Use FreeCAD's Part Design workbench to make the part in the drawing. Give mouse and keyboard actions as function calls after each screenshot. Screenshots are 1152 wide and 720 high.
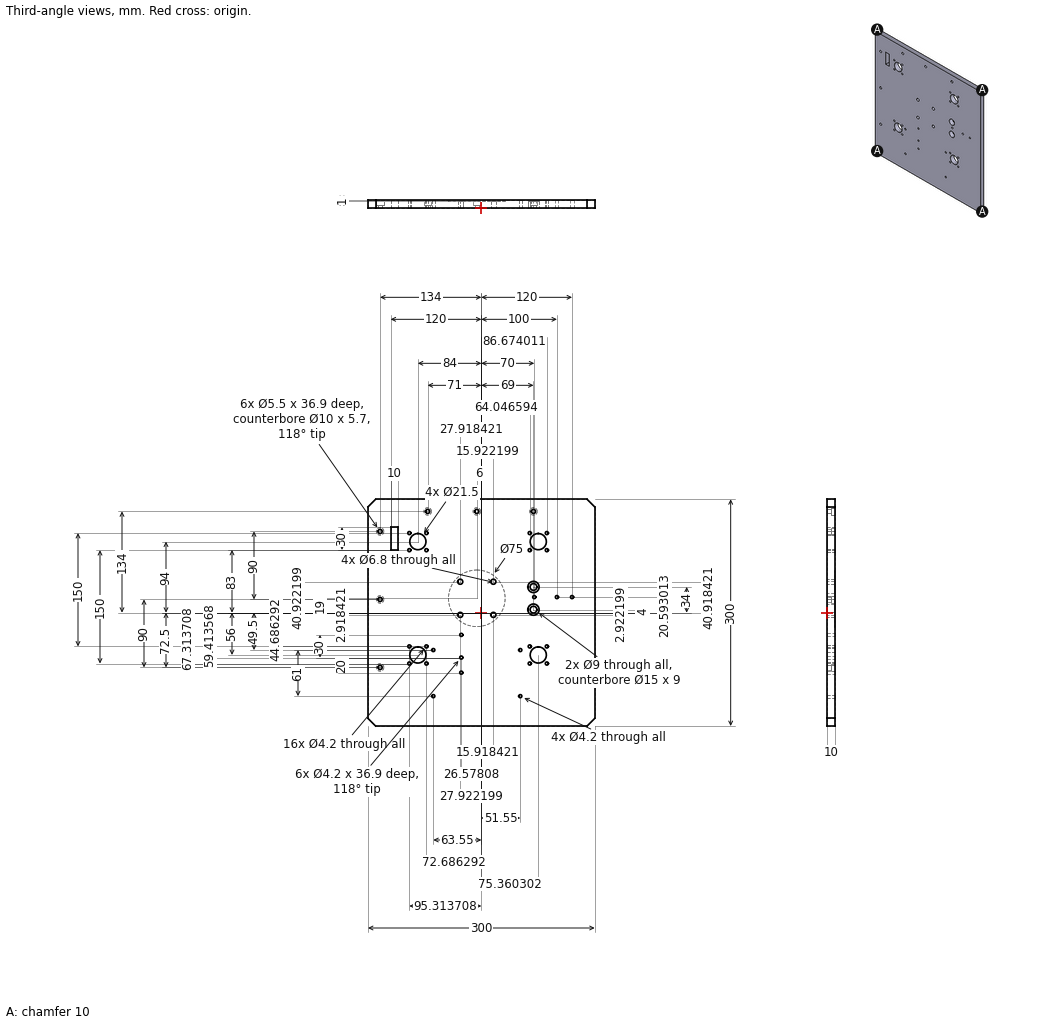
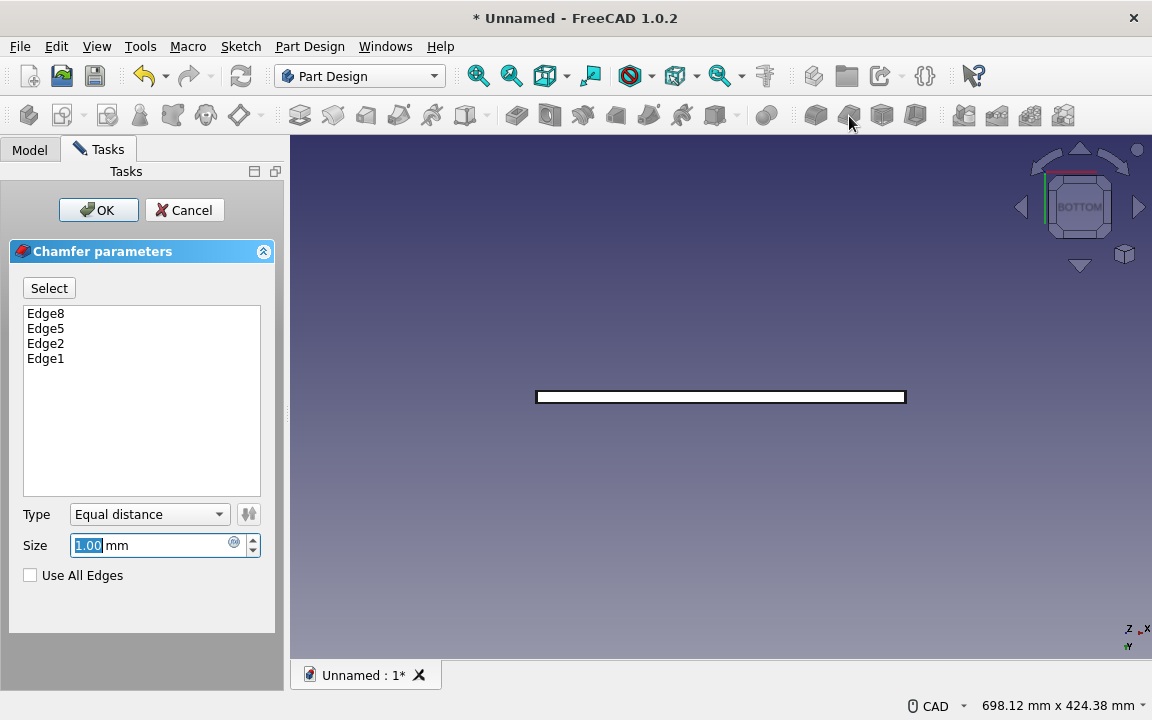
text(10)
key(Tab)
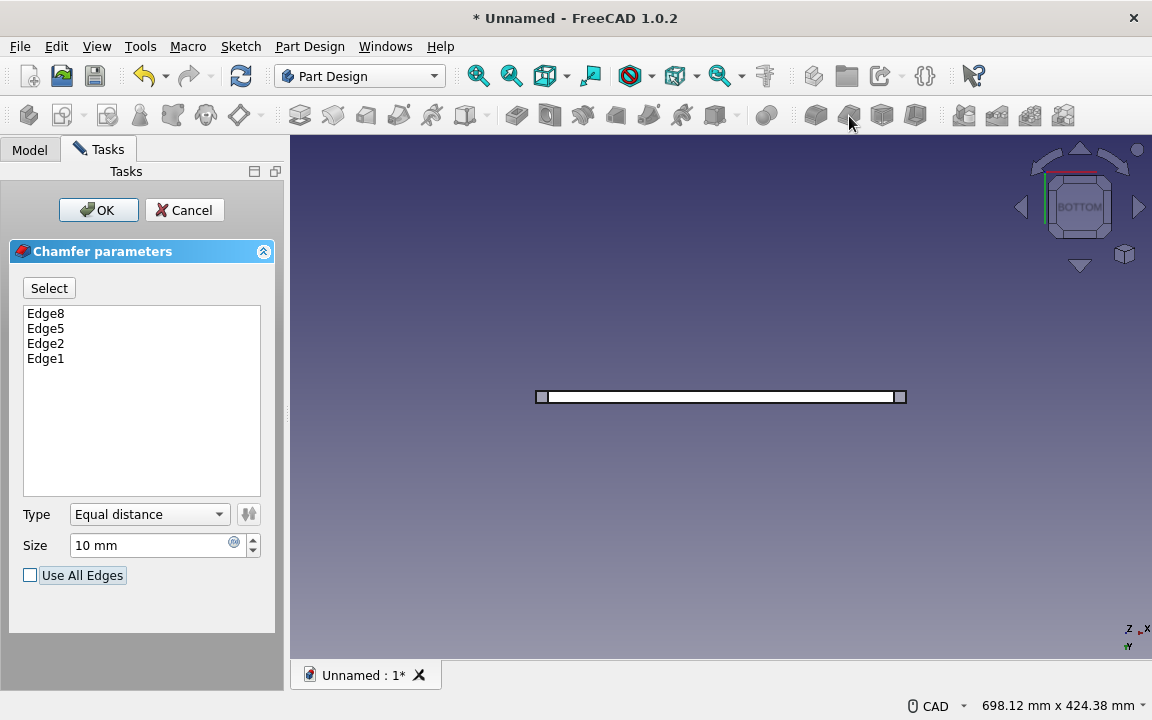
click(99, 210)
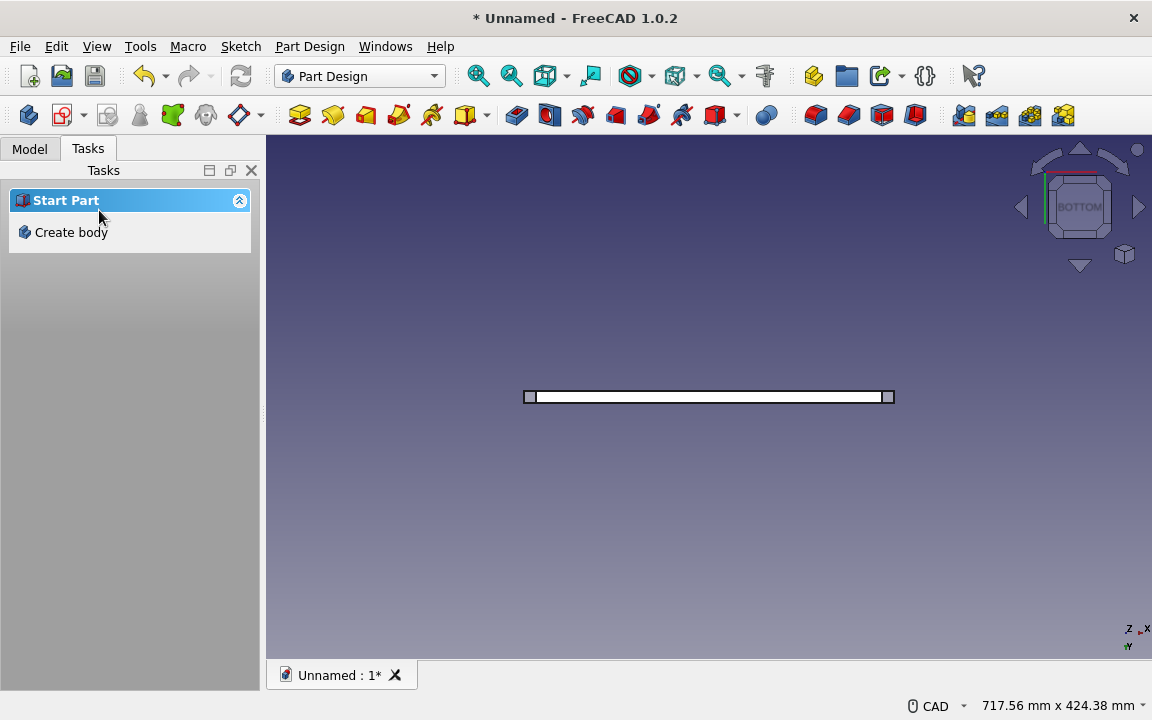
click(479, 76)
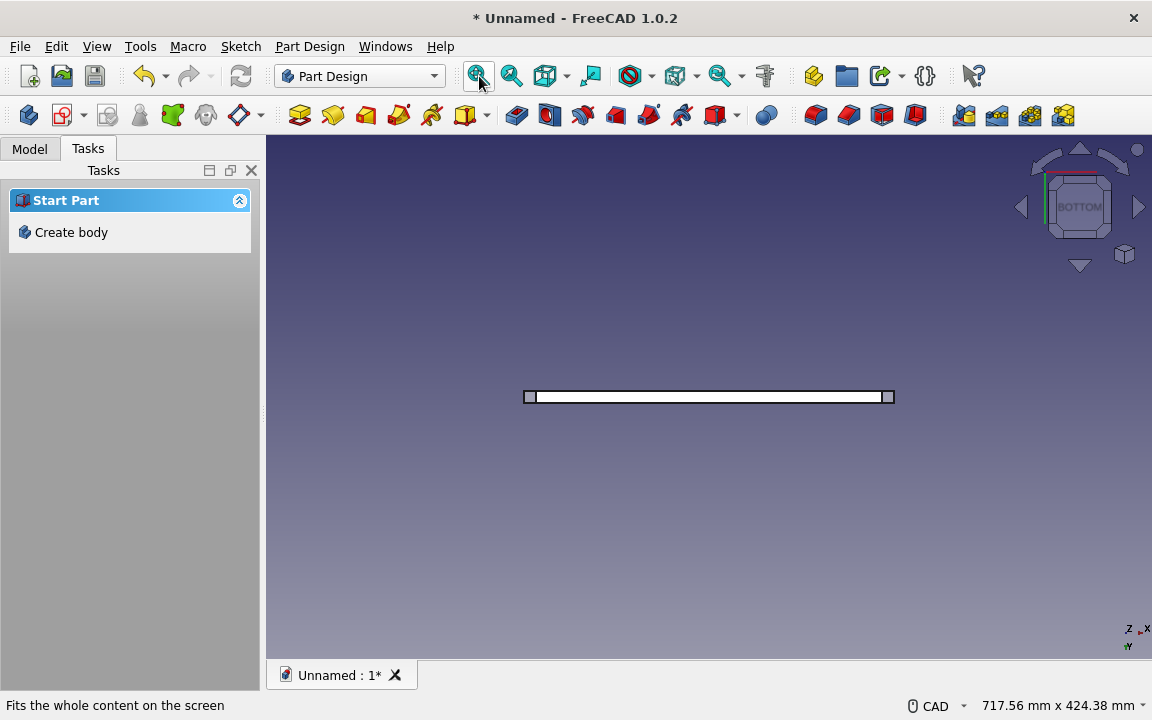
key(0)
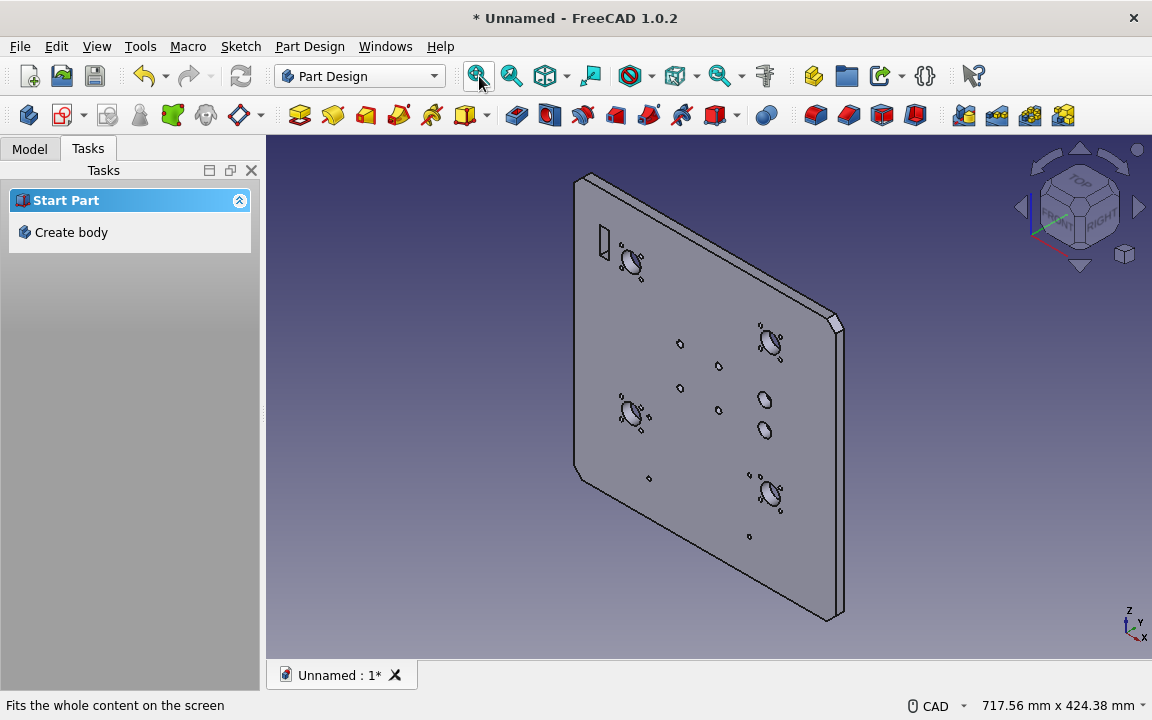
click(705, 485)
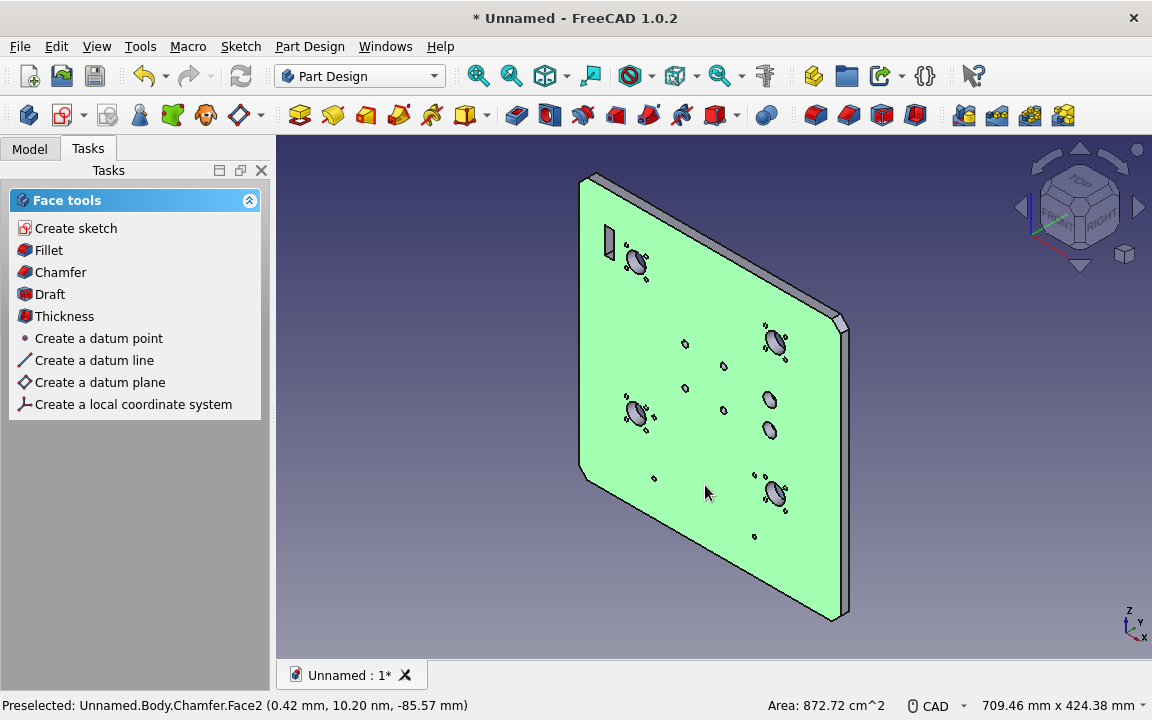
click(62, 116)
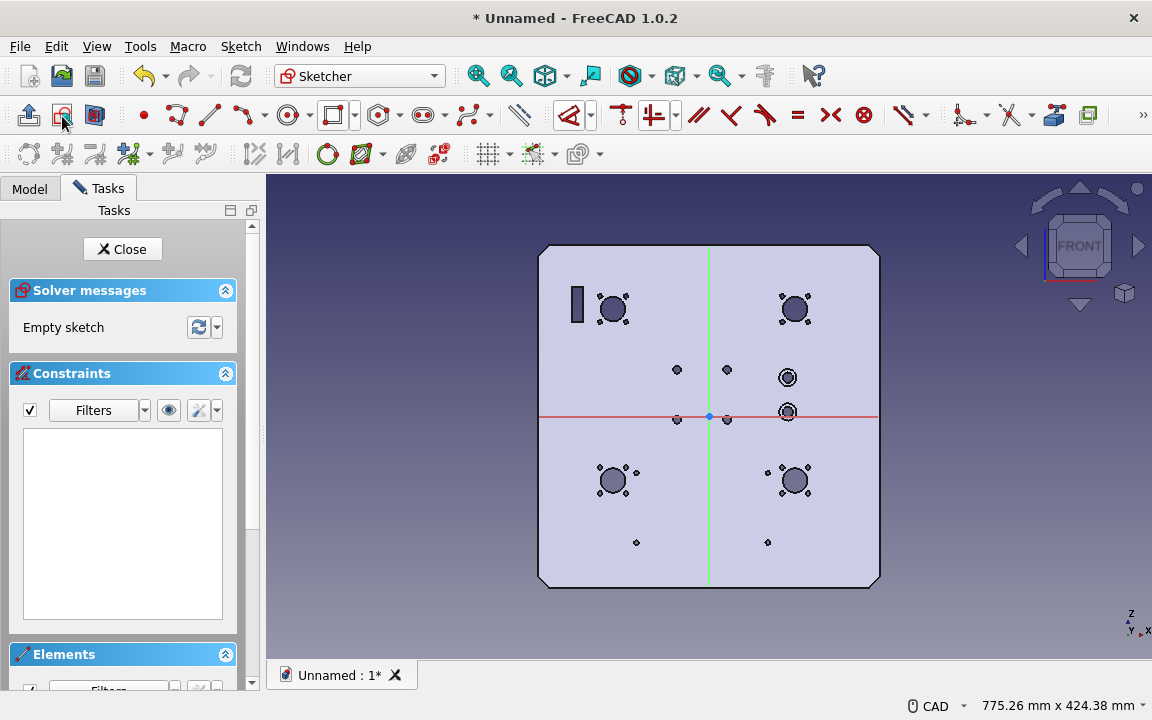
scroll(833, 470, up, 5)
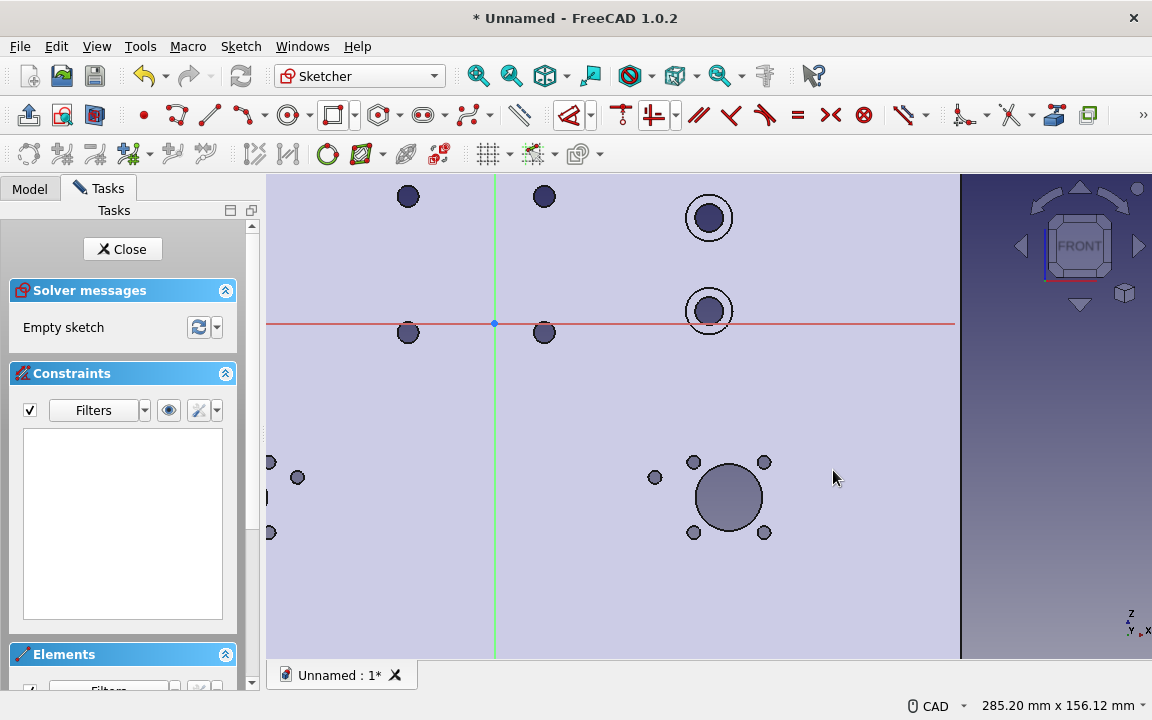
key(g)
key(c)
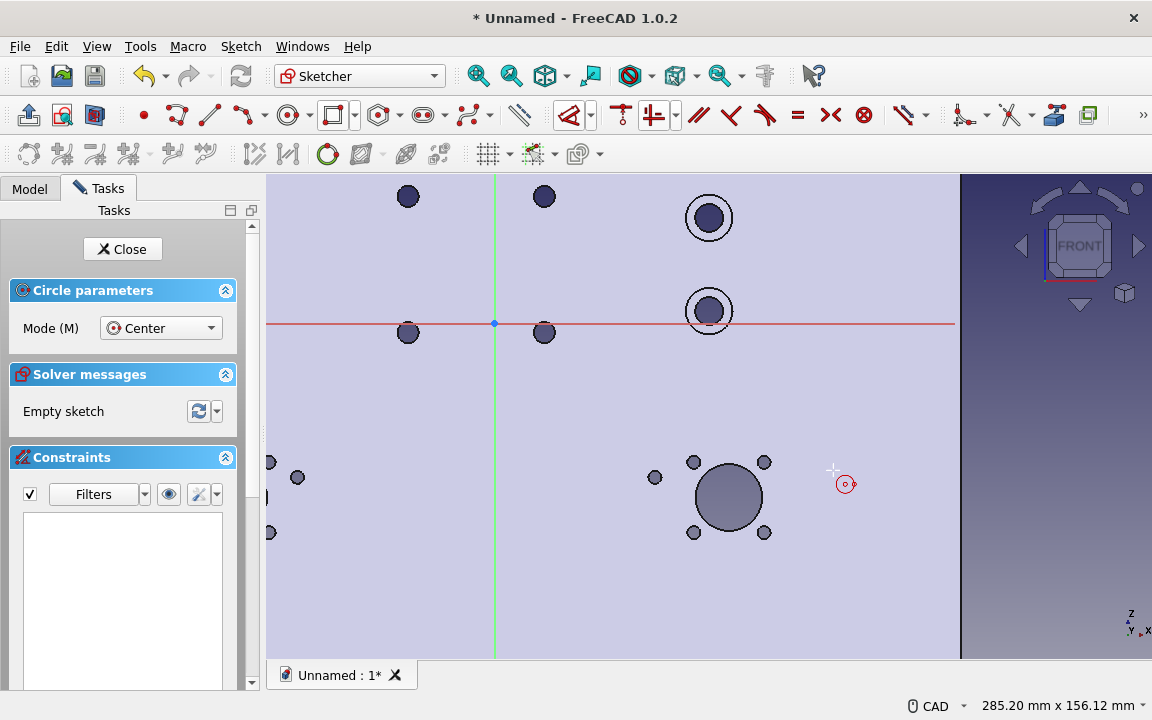
scroll(412, 508, up, 7)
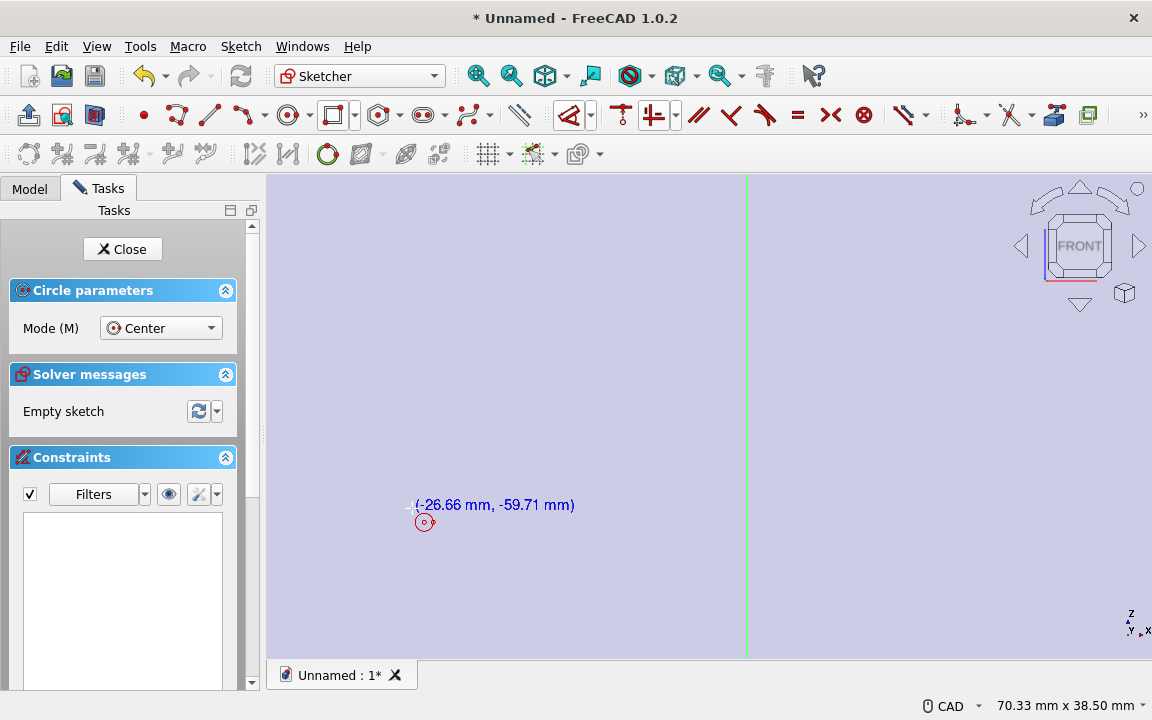
scroll(413, 511, down, 7)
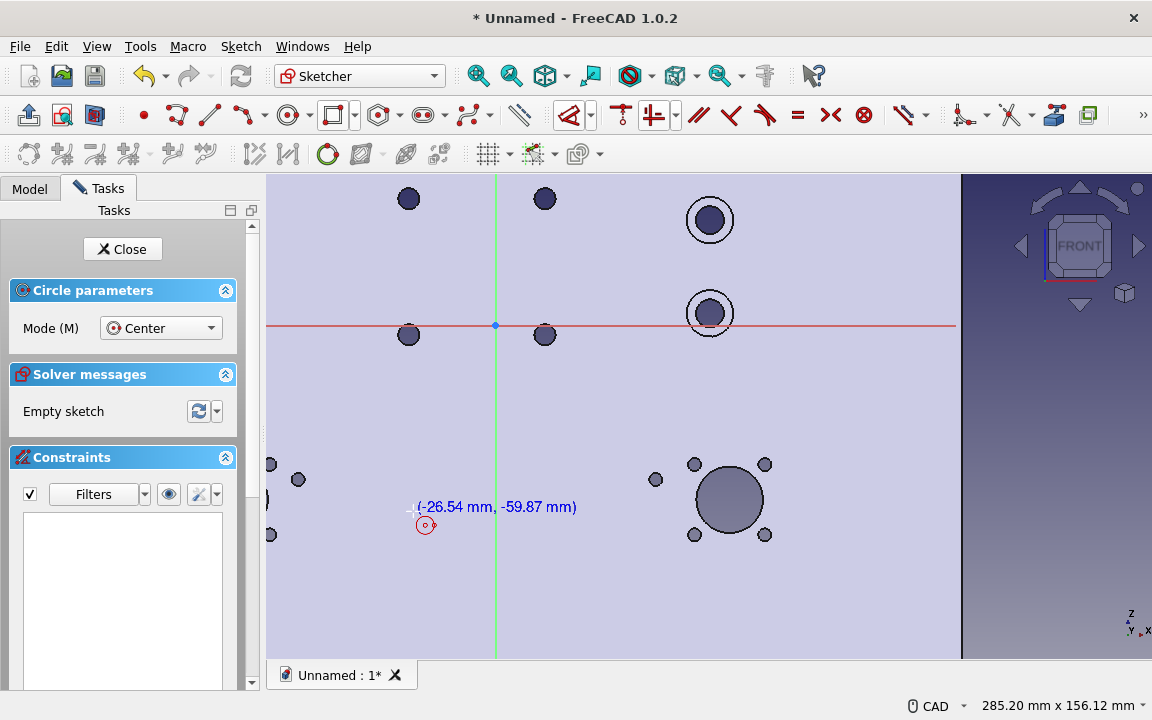
click(413, 510)
move(418, 506)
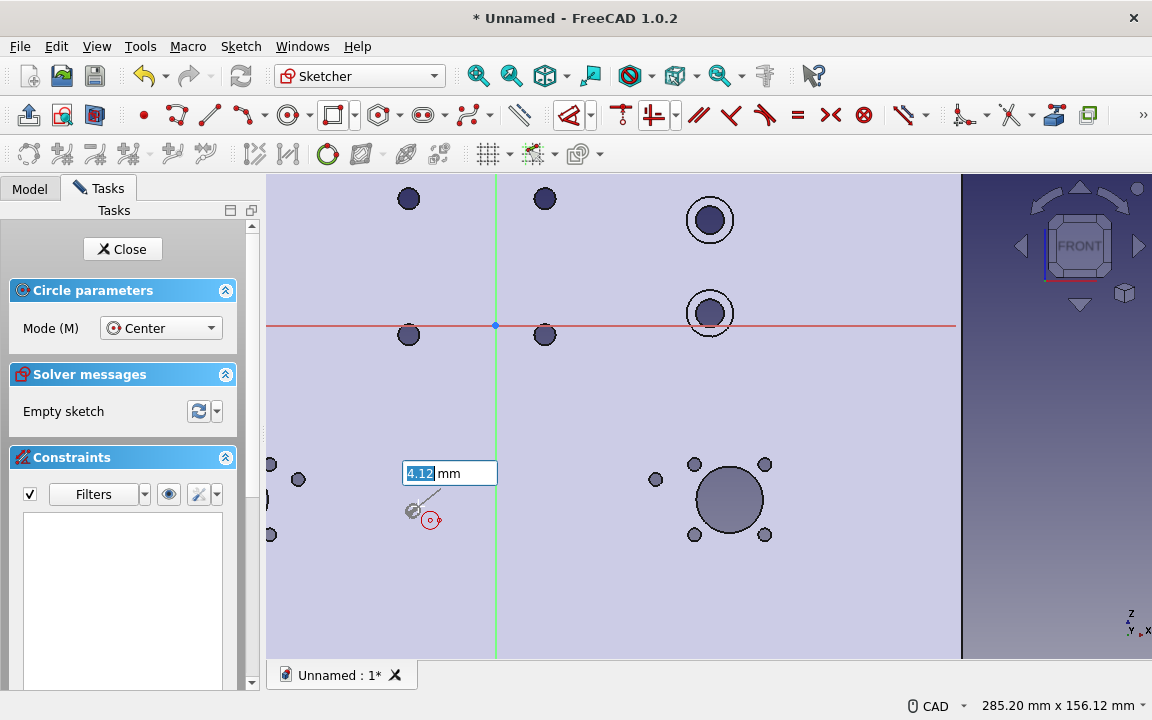
text(4.2)
key(Return)